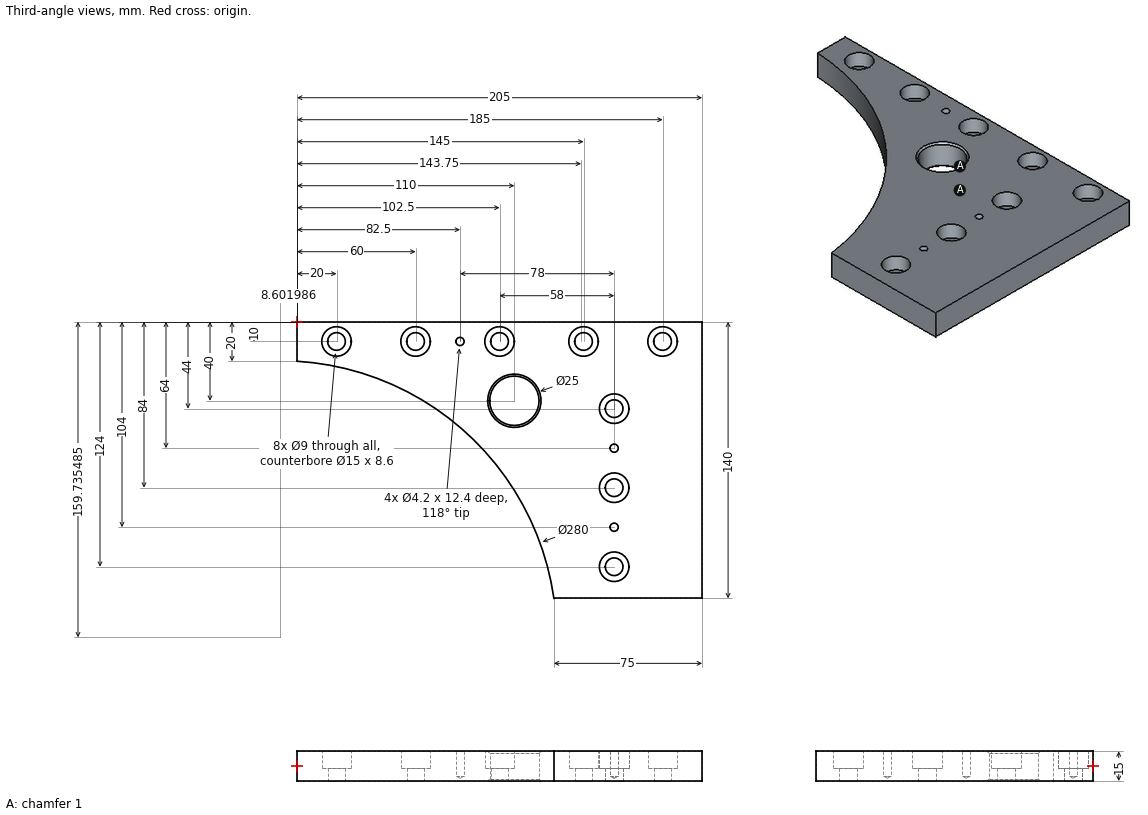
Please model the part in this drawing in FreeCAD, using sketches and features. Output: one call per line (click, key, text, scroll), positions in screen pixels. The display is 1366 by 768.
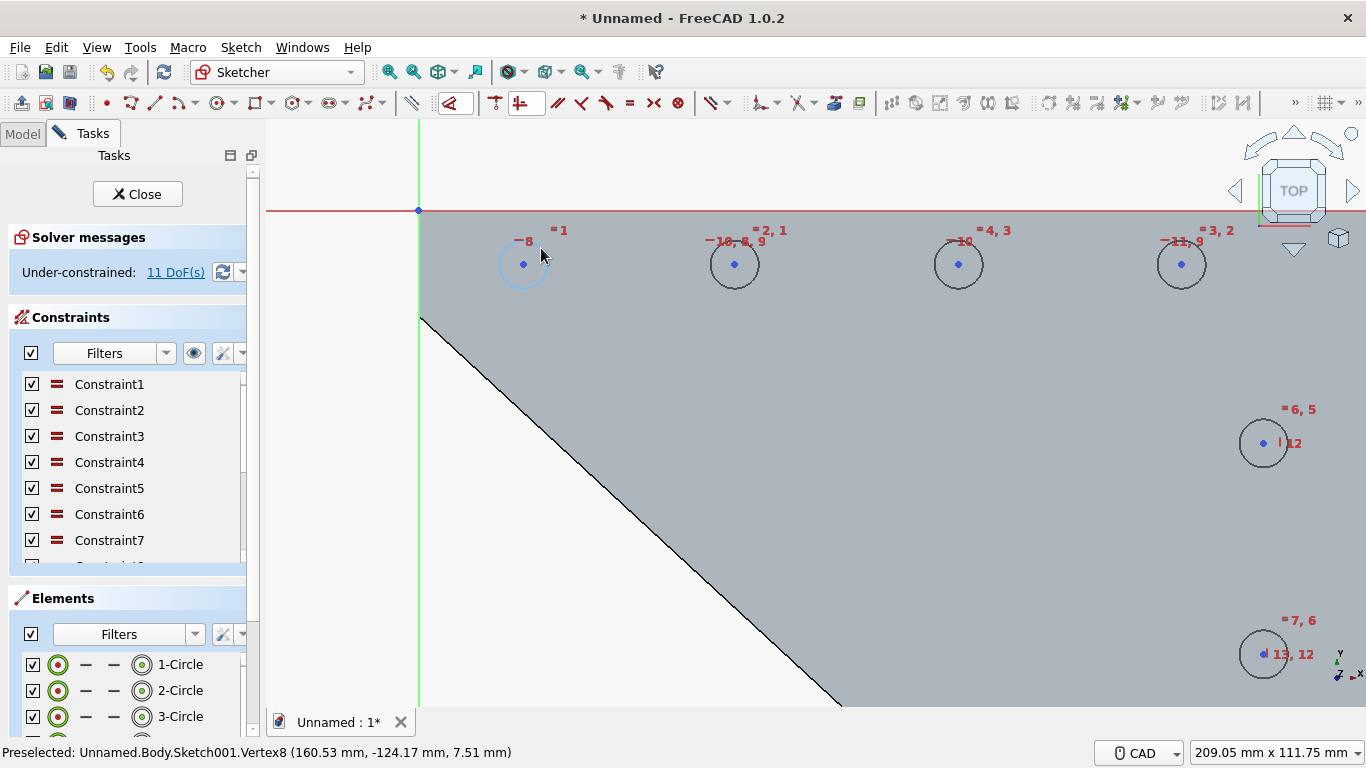
click(541, 248)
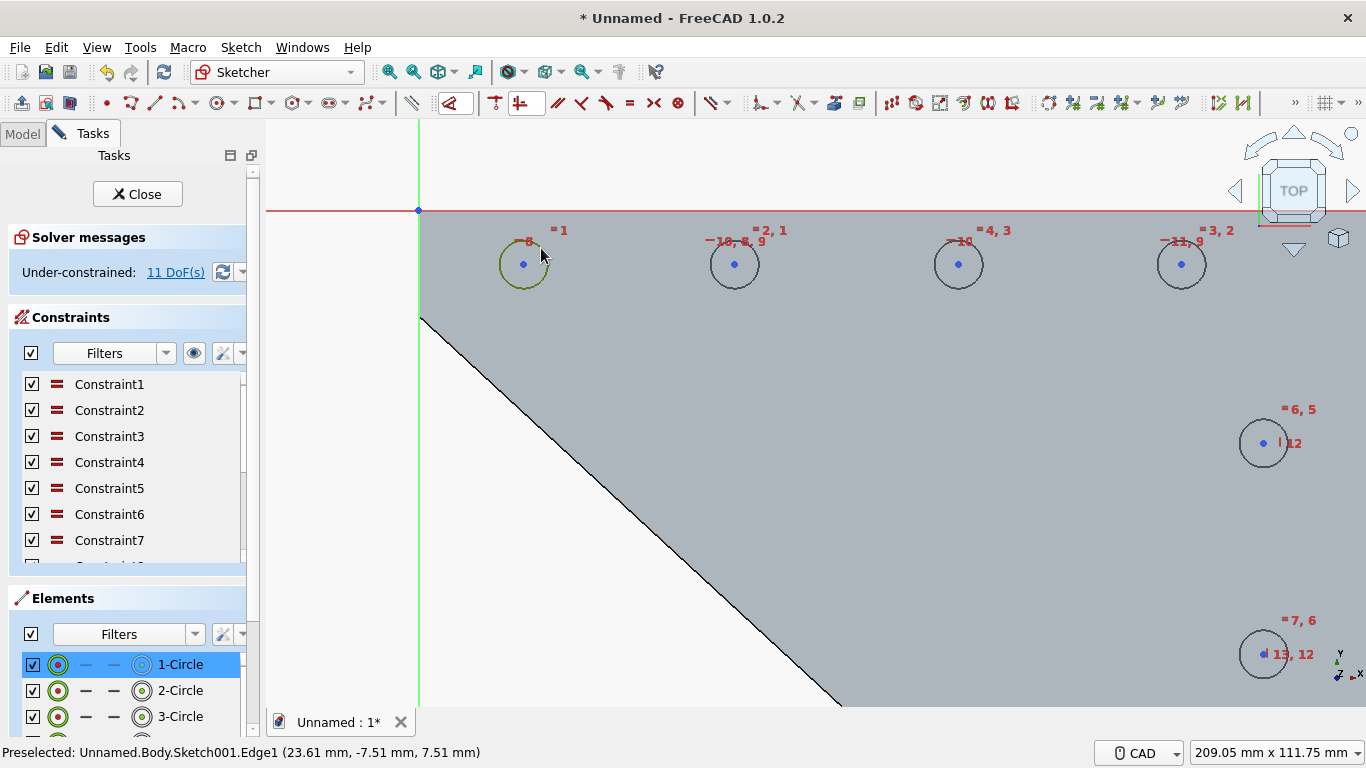
click(468, 104)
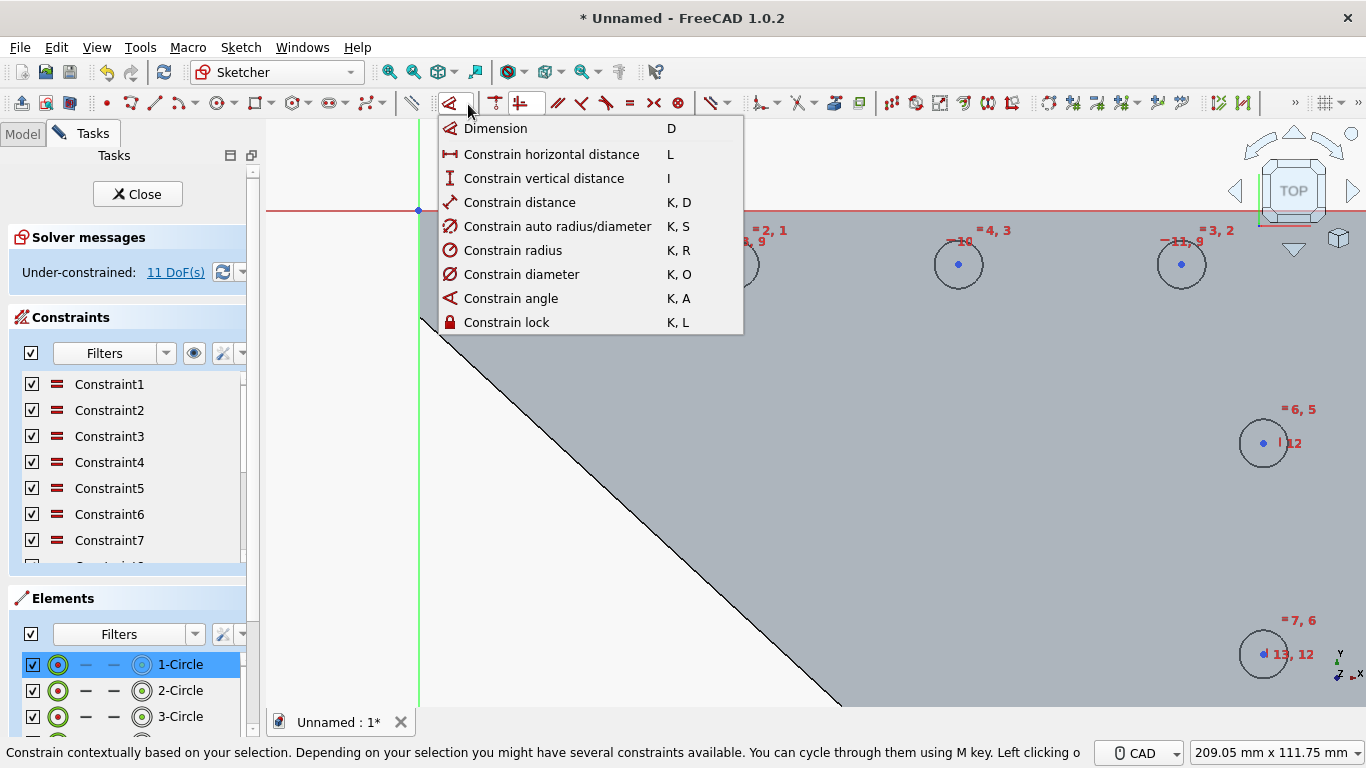
click(591, 274)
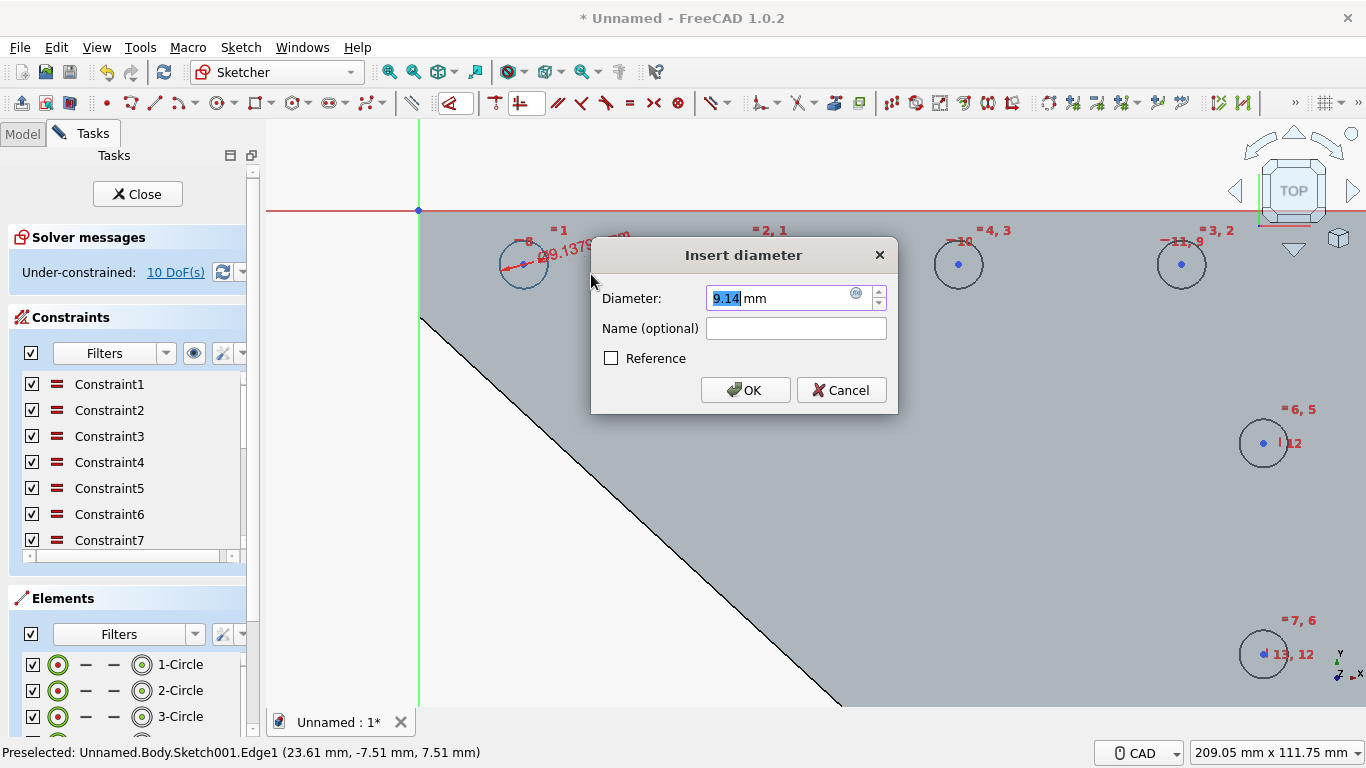
text(9)
key(Return)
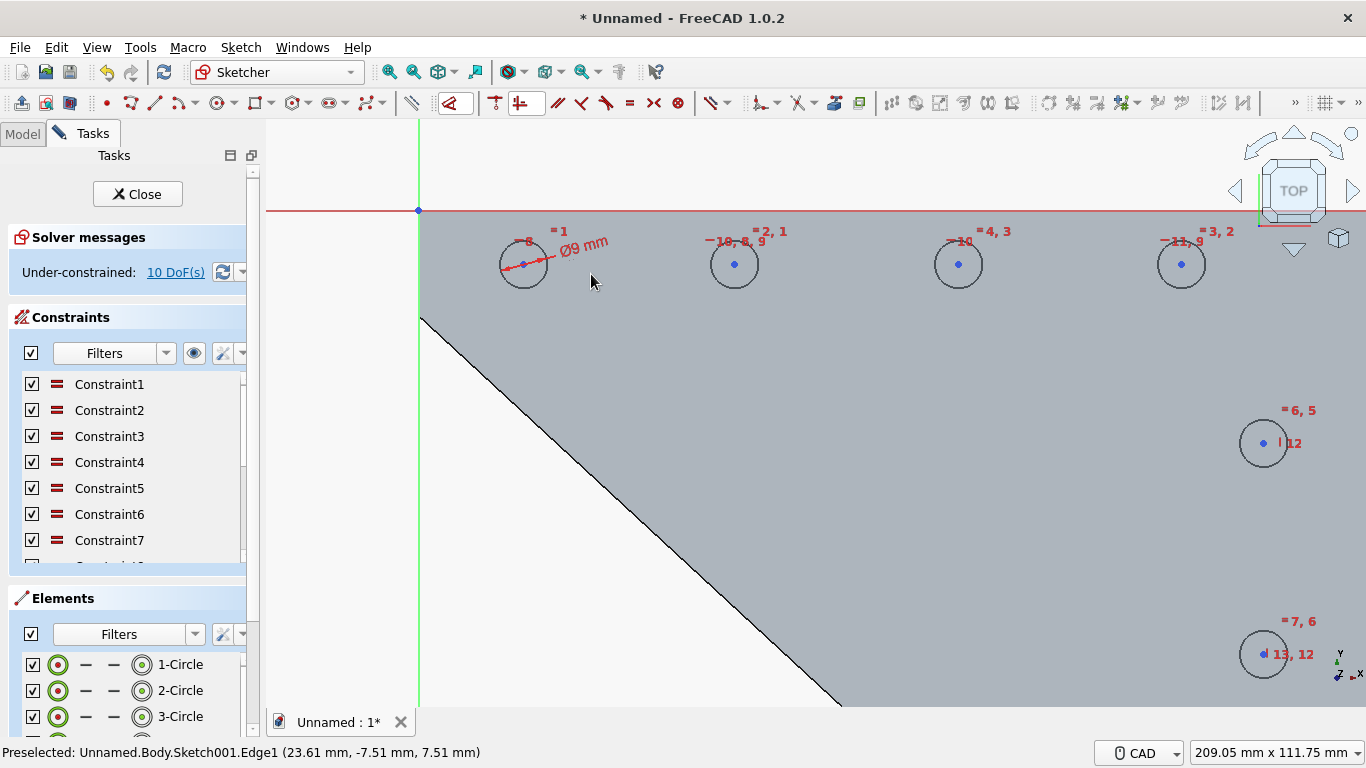
click(524, 265)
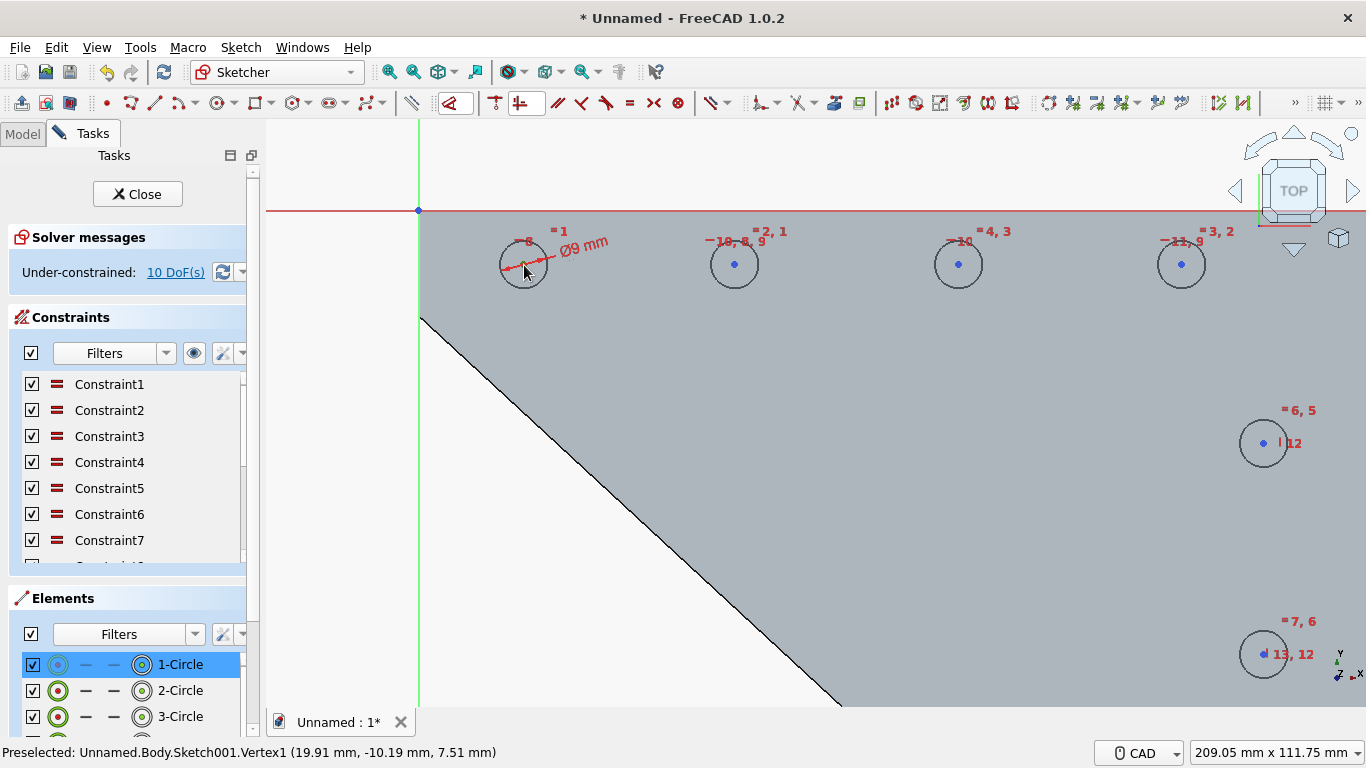
click(468, 104)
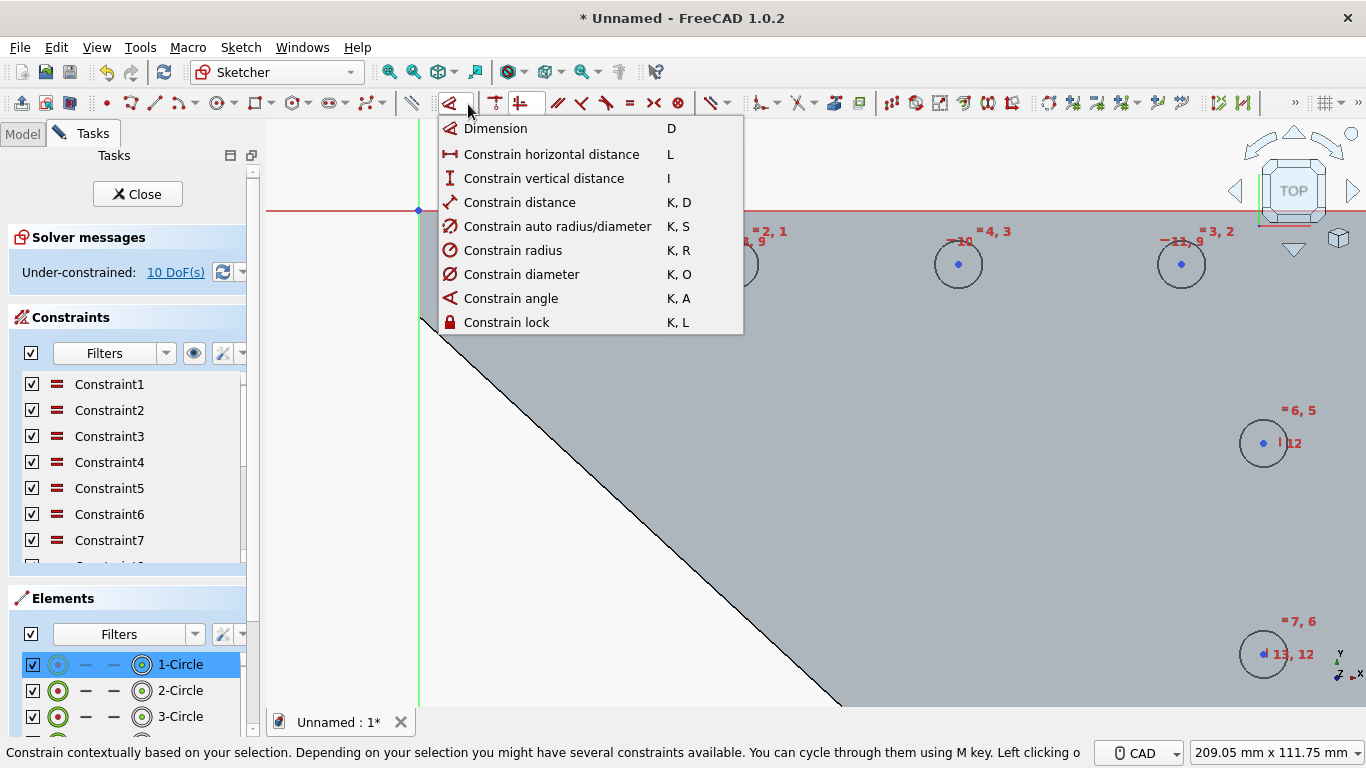
click(591, 154)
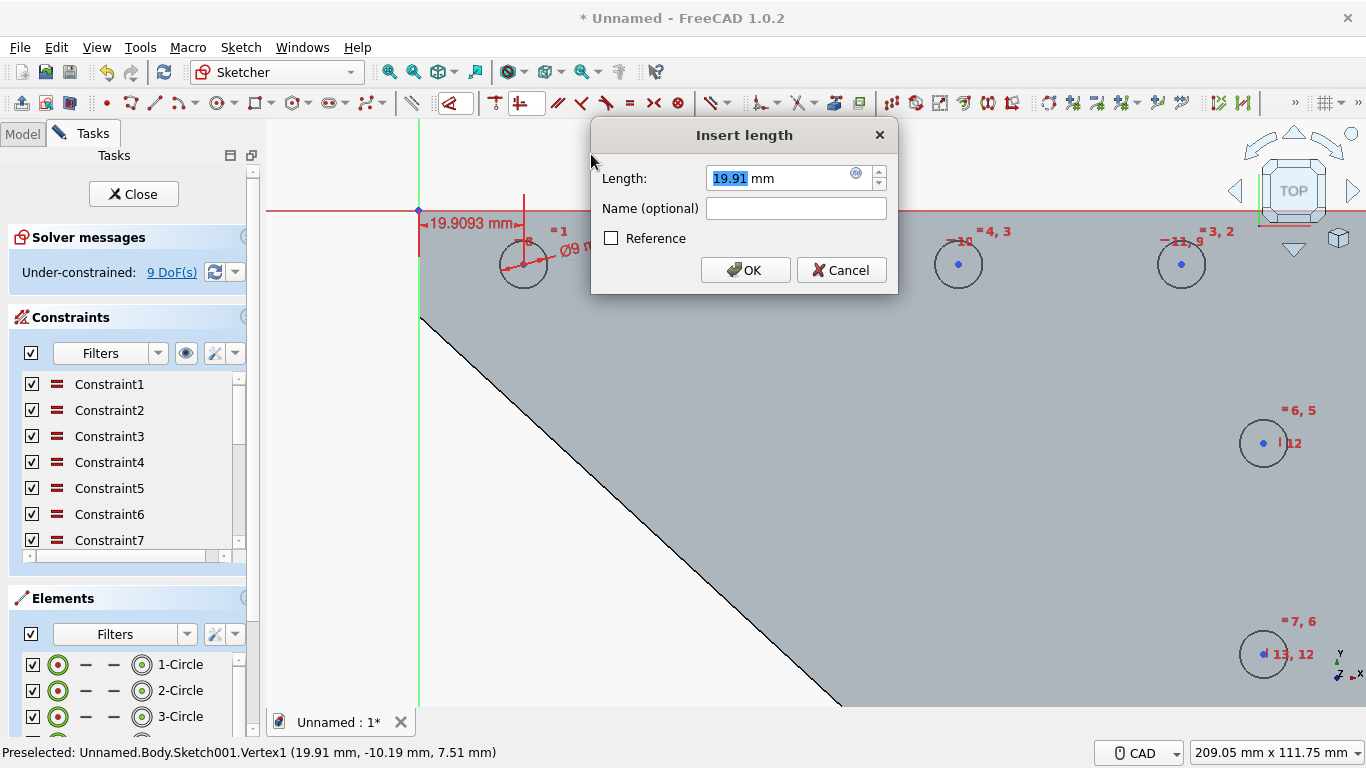
text(20)
key(Return)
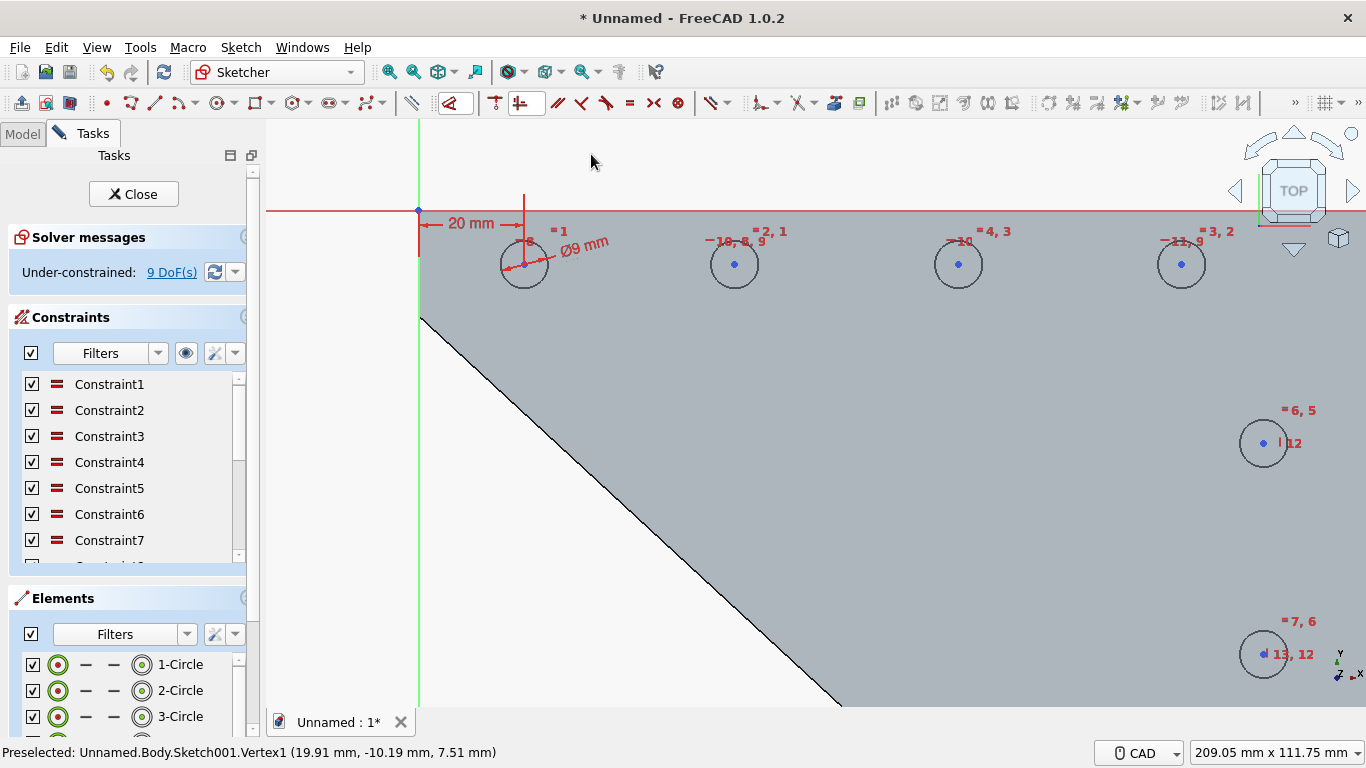
click(524, 265)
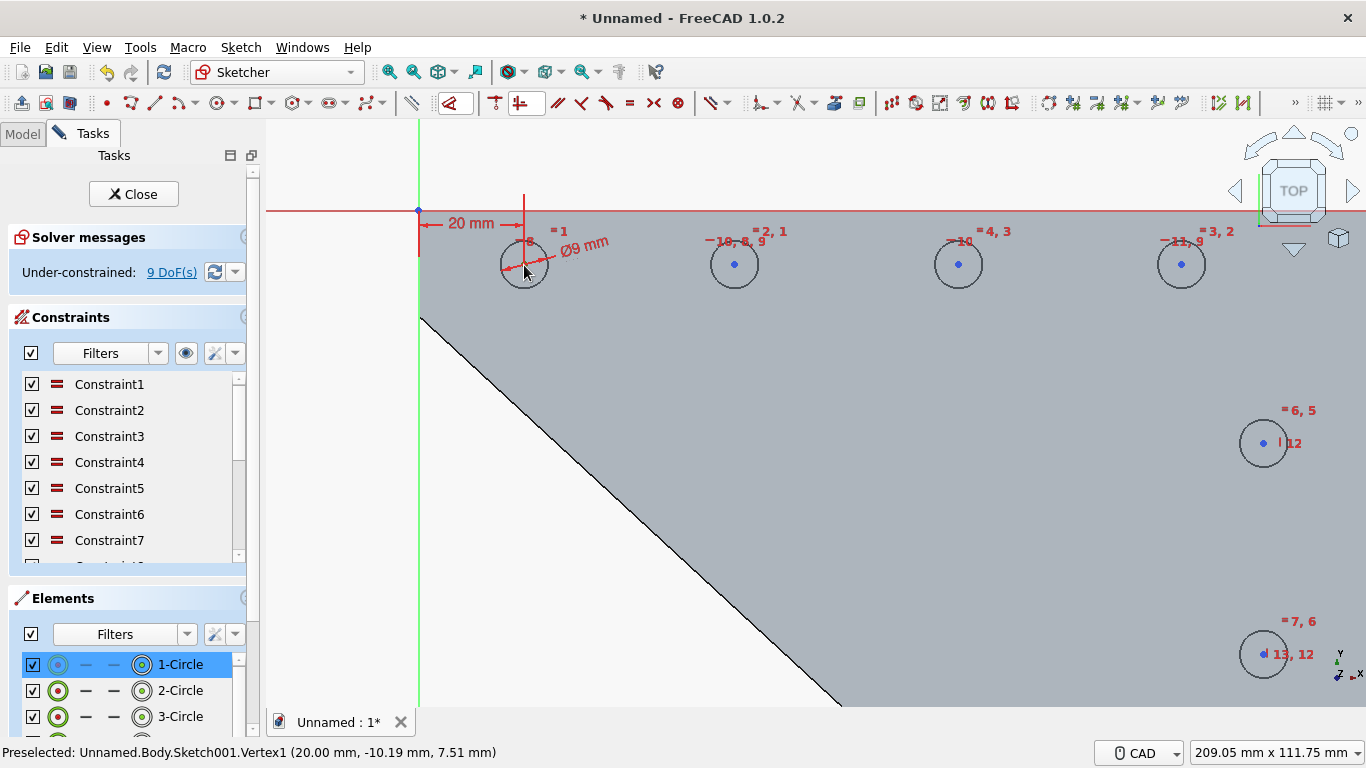
click(468, 104)